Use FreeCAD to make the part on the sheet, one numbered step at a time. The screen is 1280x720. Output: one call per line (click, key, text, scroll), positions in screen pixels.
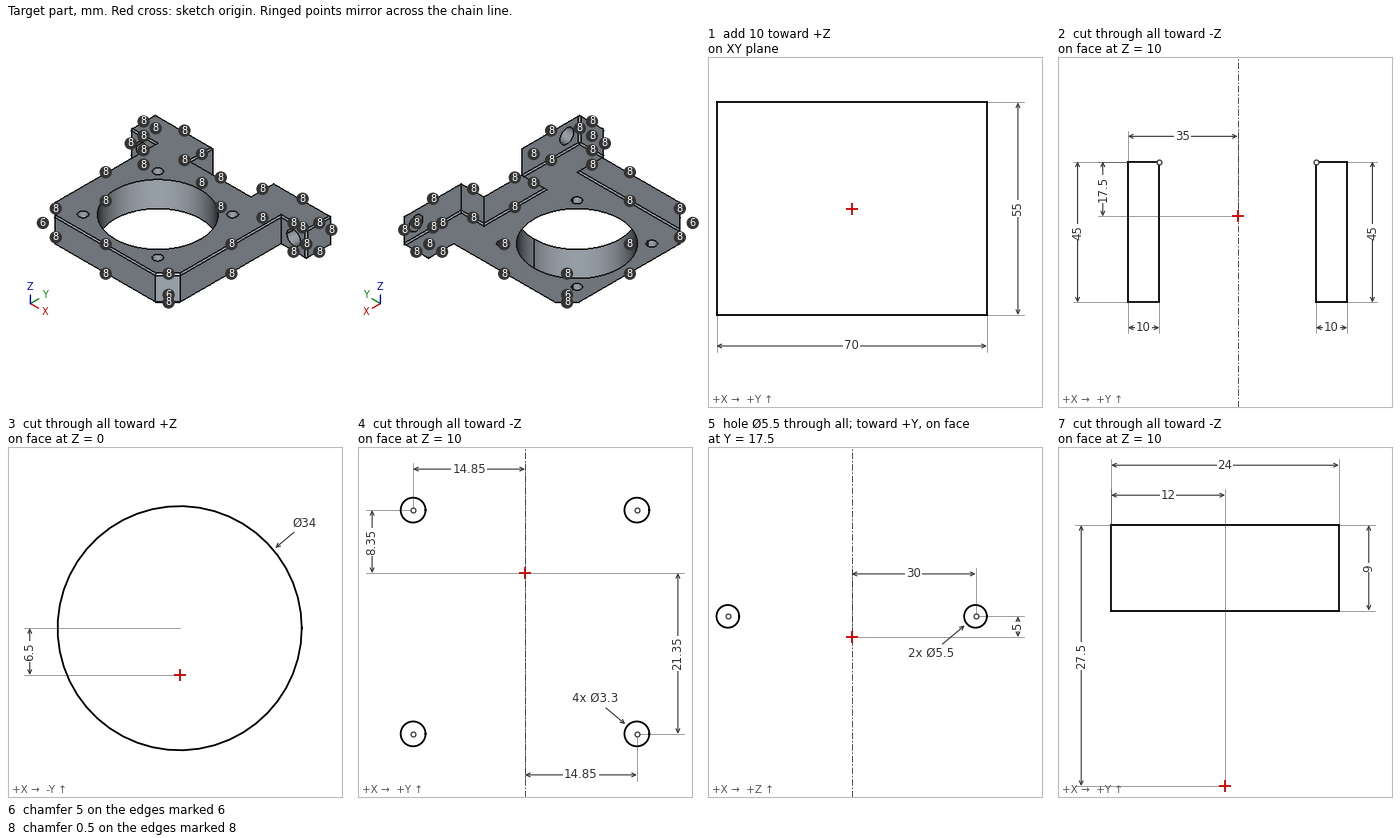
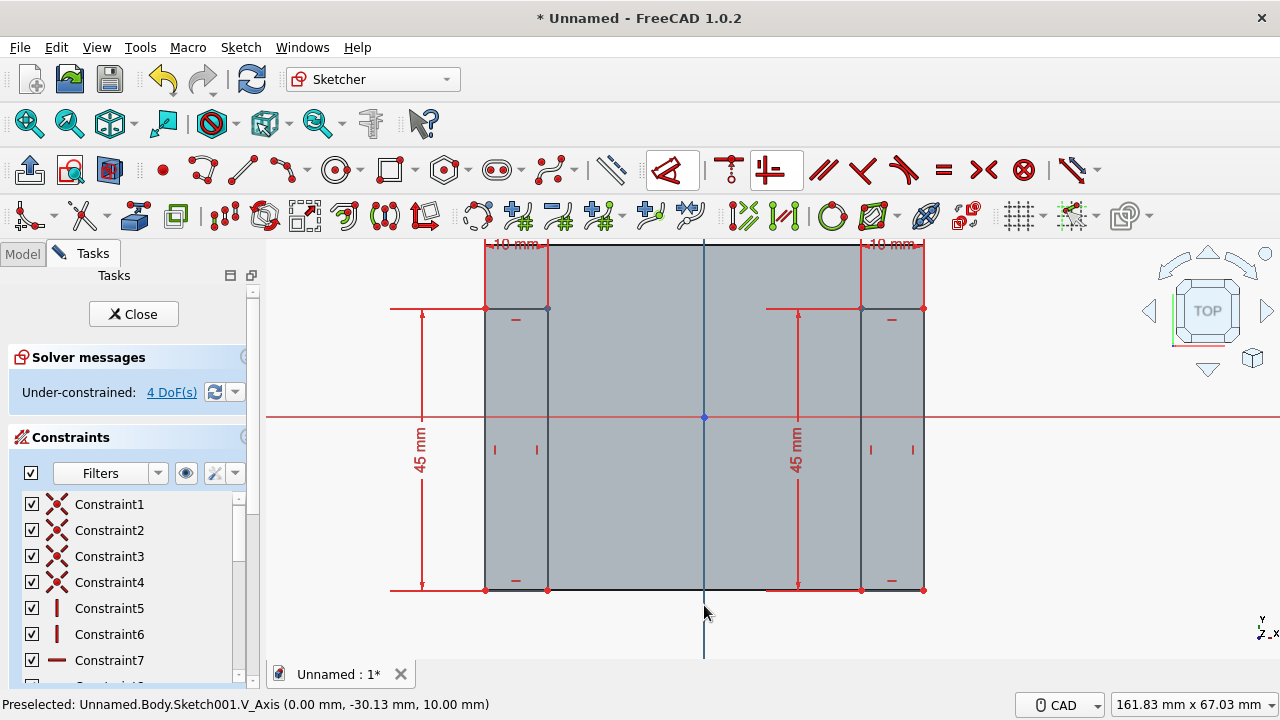
click(984, 170)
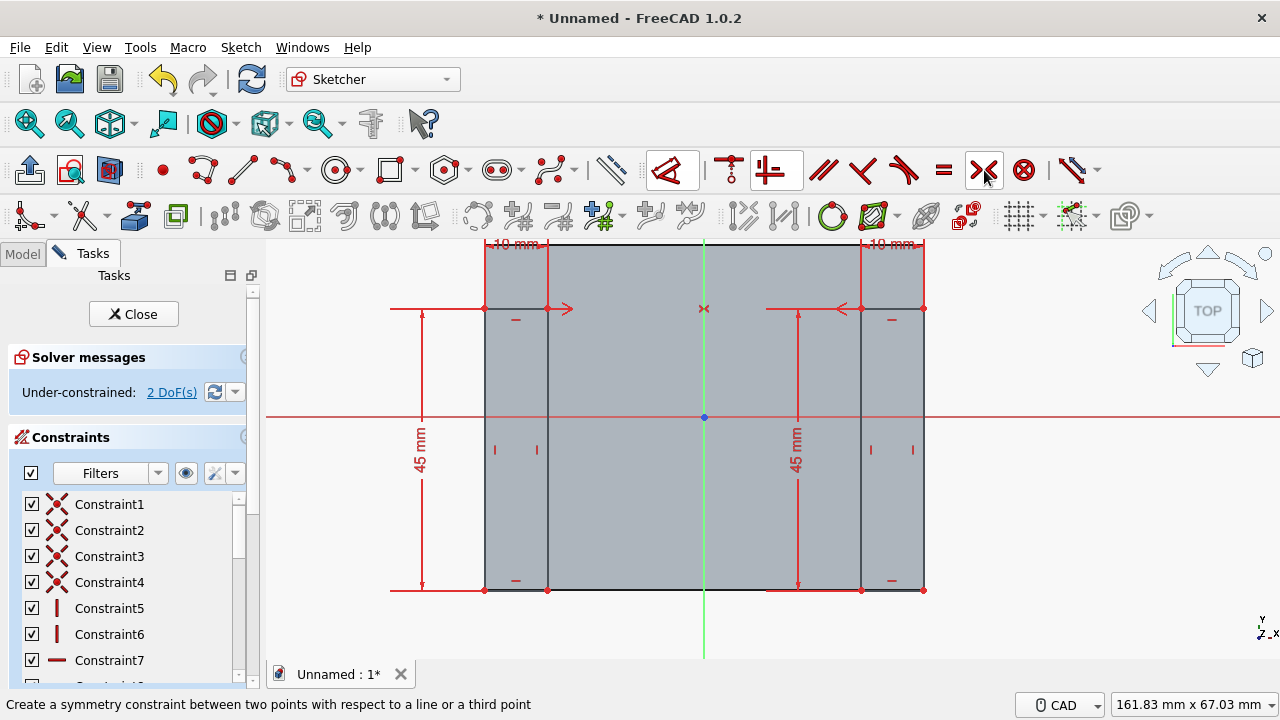
click(485, 309)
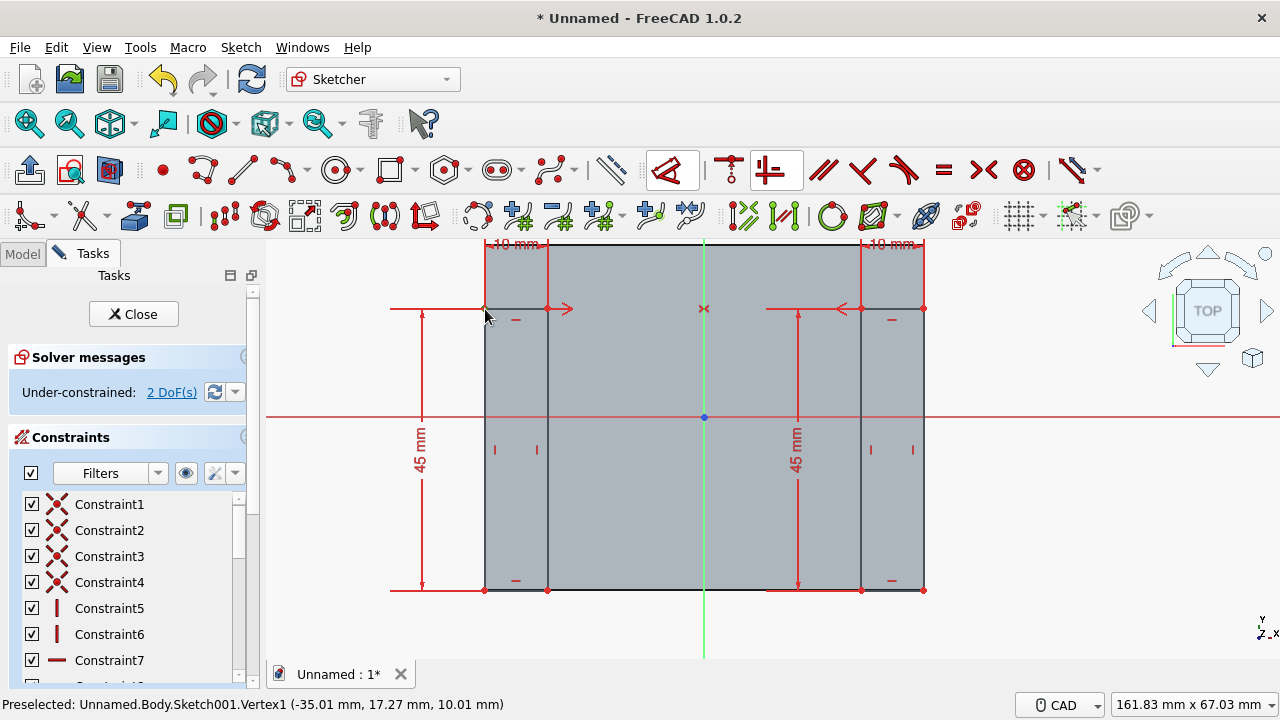
click(694, 170)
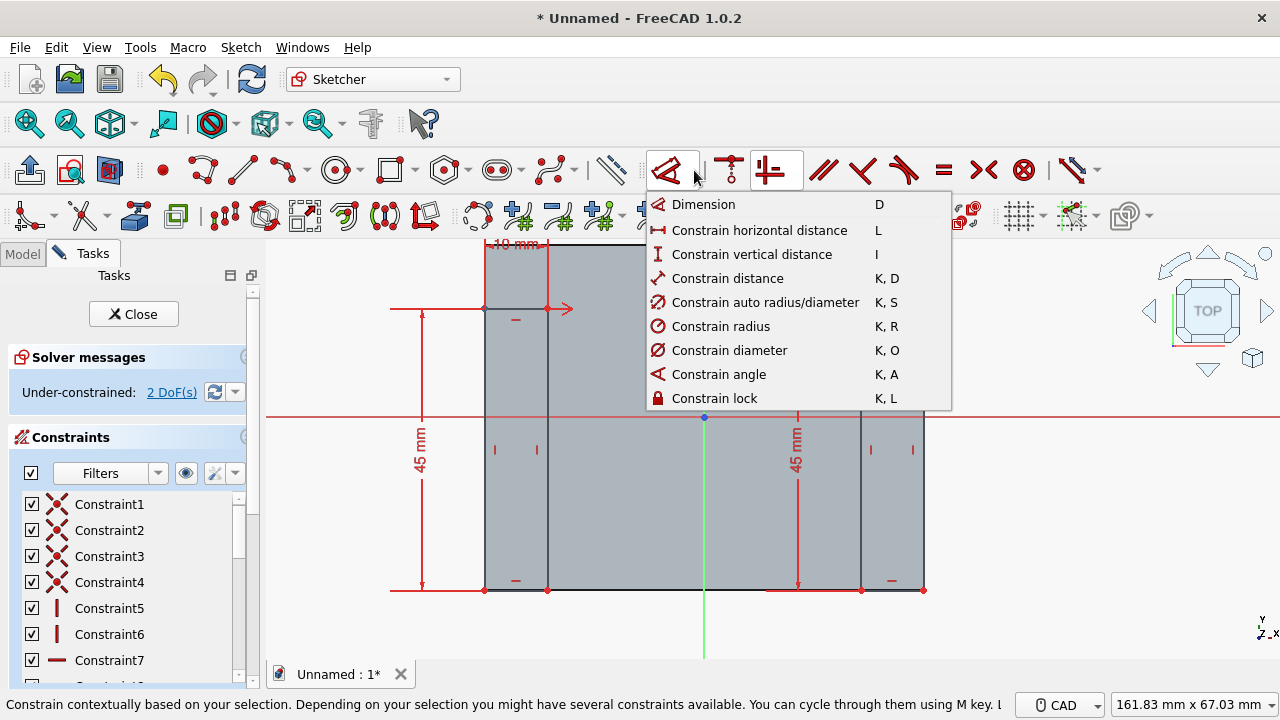
click(799, 230)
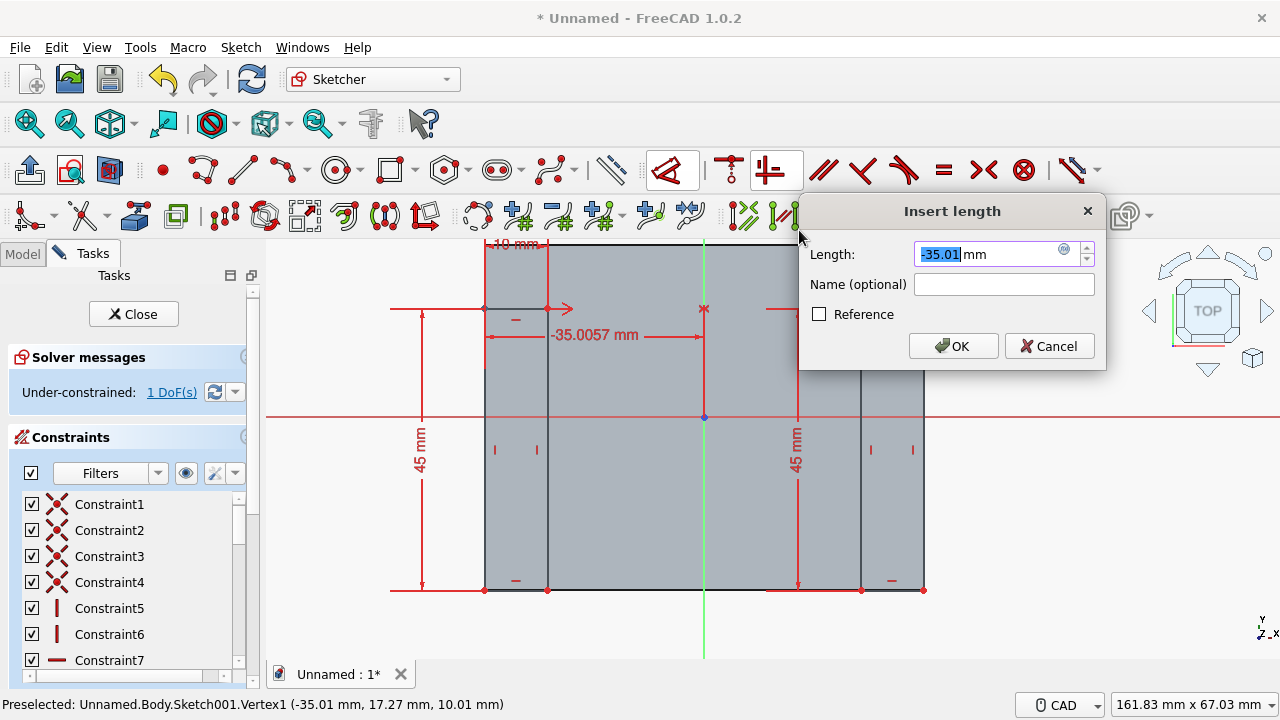
text(-35)
key(Return)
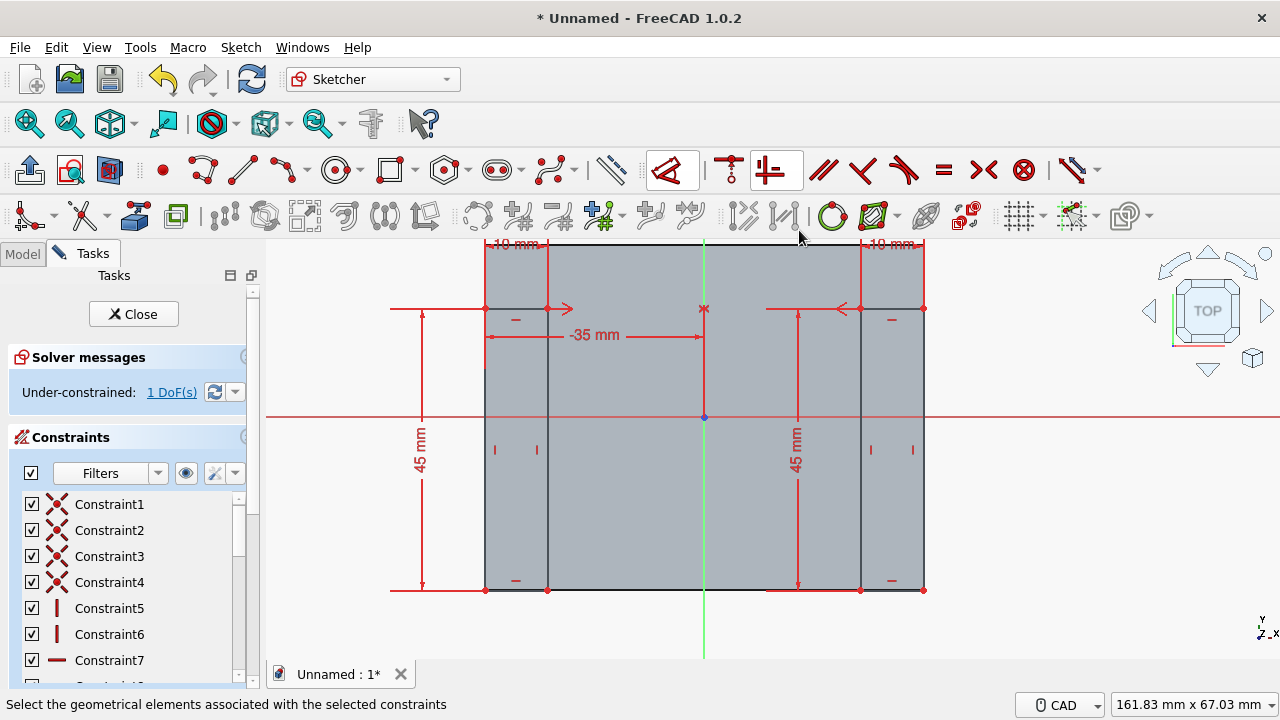
click(485, 309)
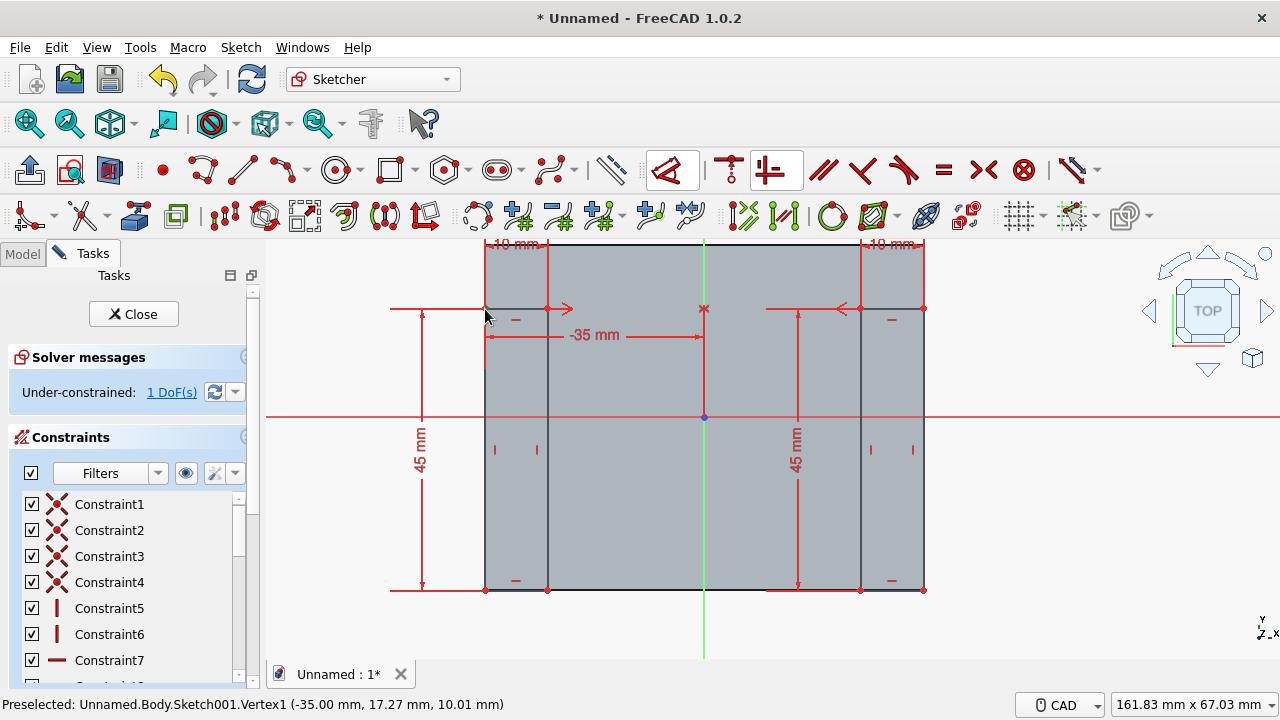
key(i)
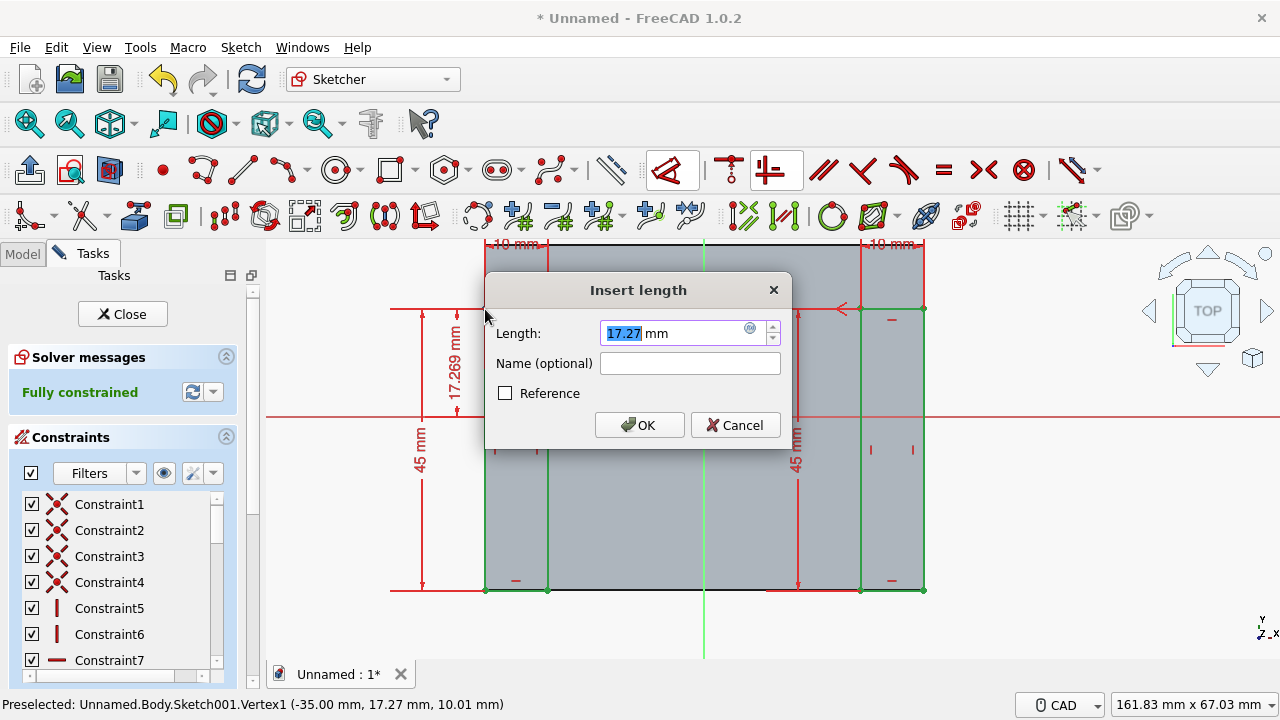
text(17.5)
key(Return)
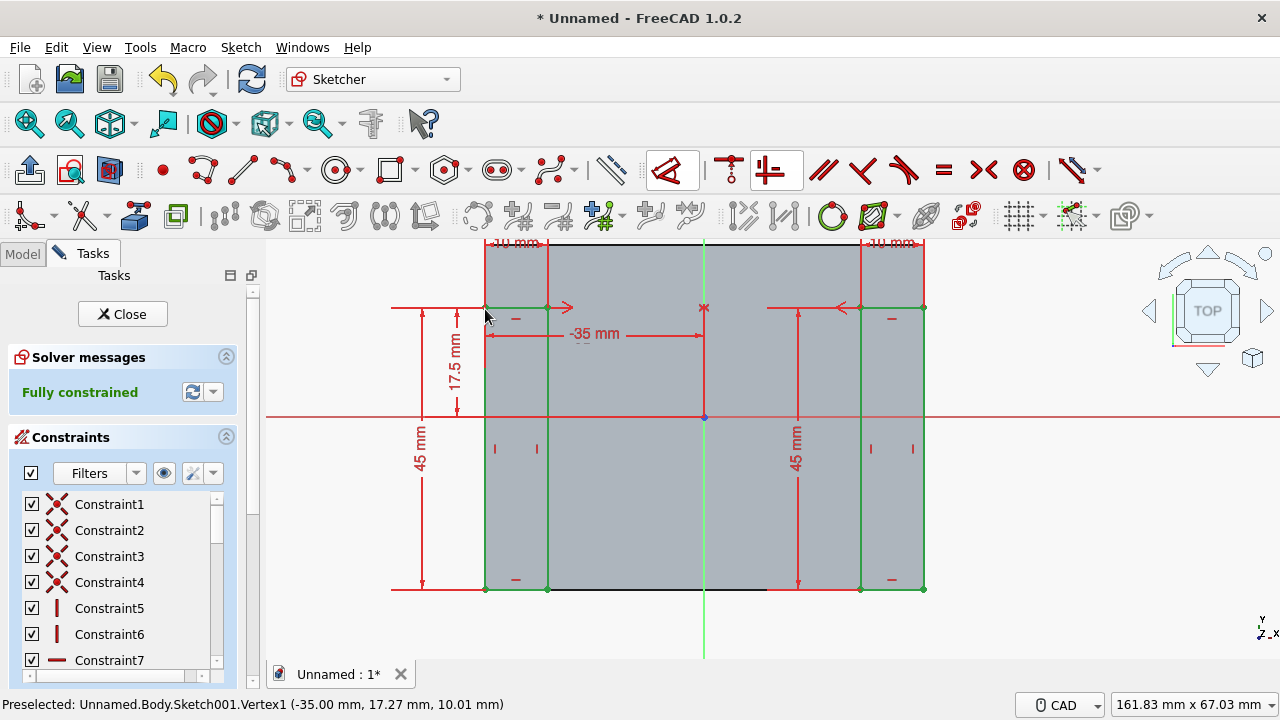
click(123, 314)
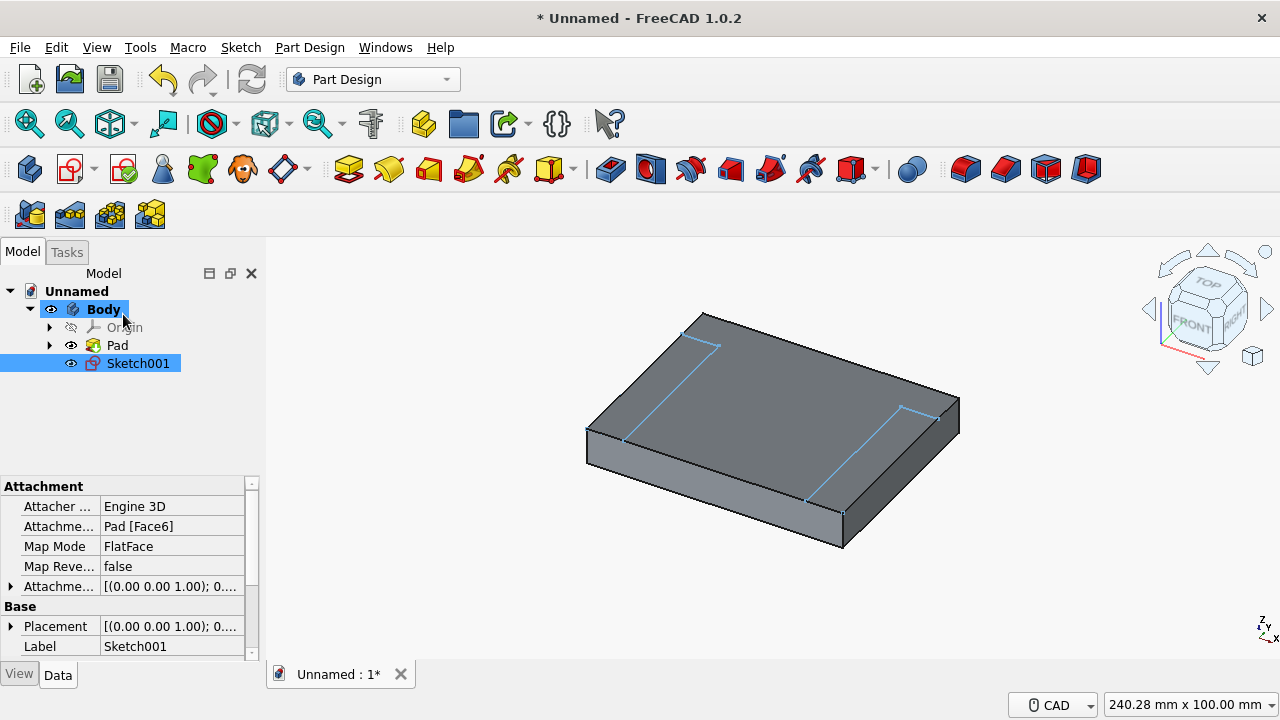
click(612, 170)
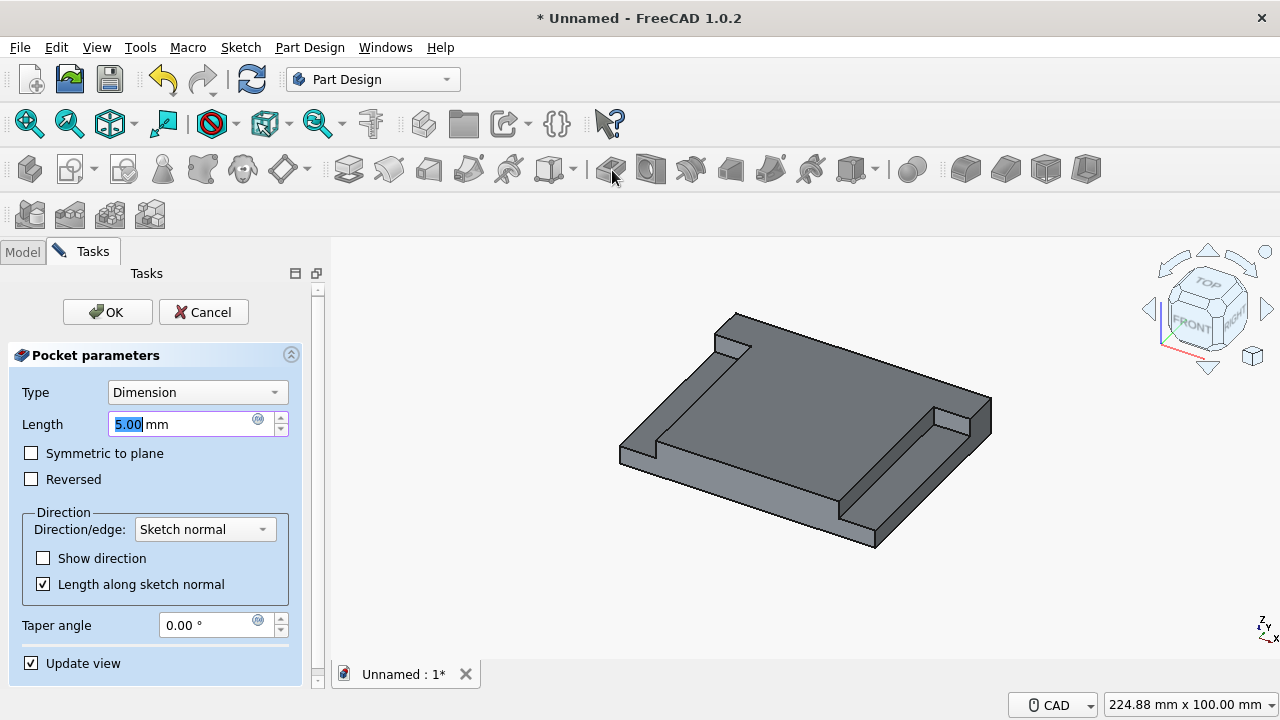
click(198, 392)